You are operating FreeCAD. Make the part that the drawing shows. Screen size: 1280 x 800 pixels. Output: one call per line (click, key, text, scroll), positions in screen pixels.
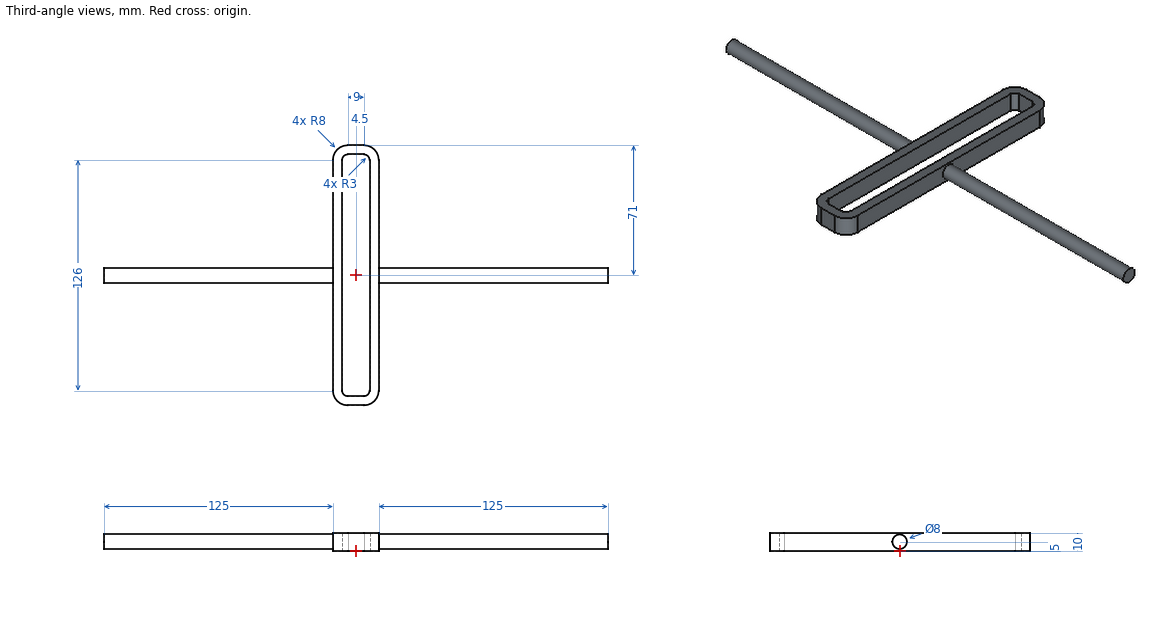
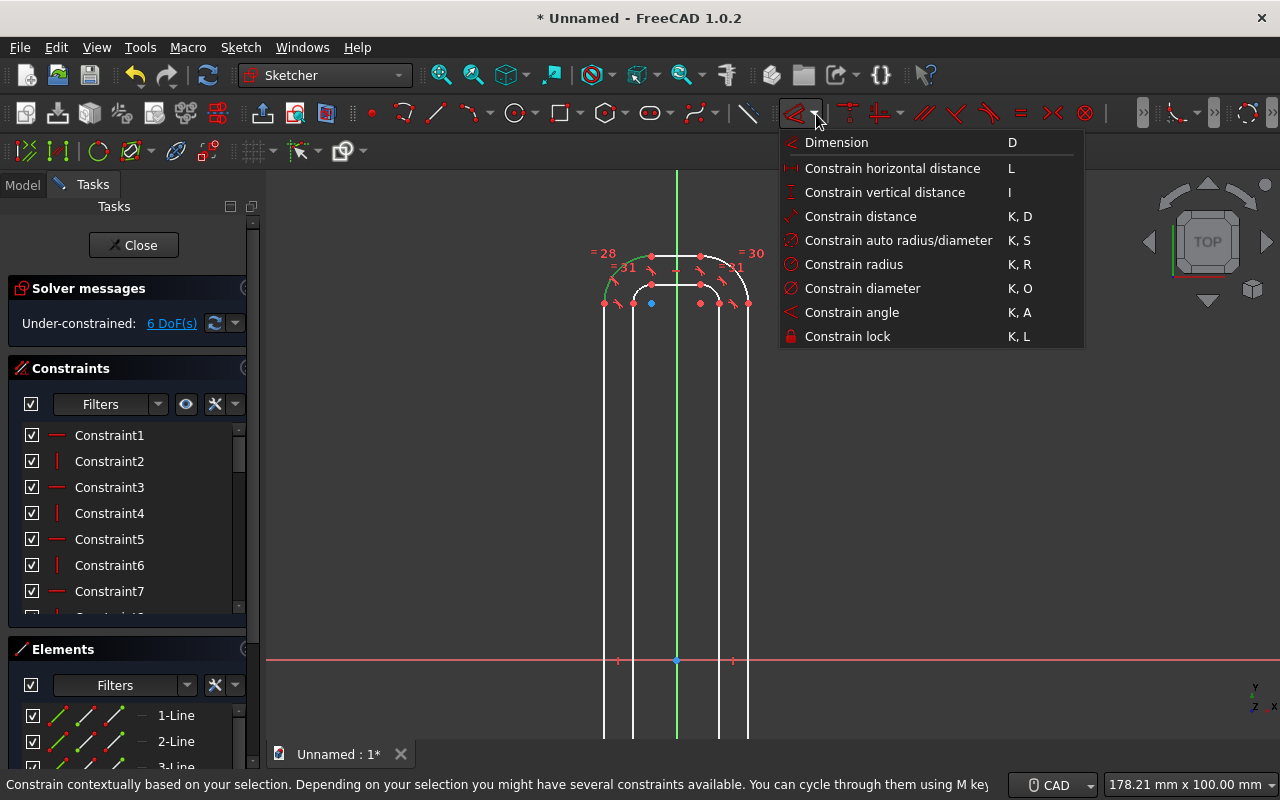
click(932, 264)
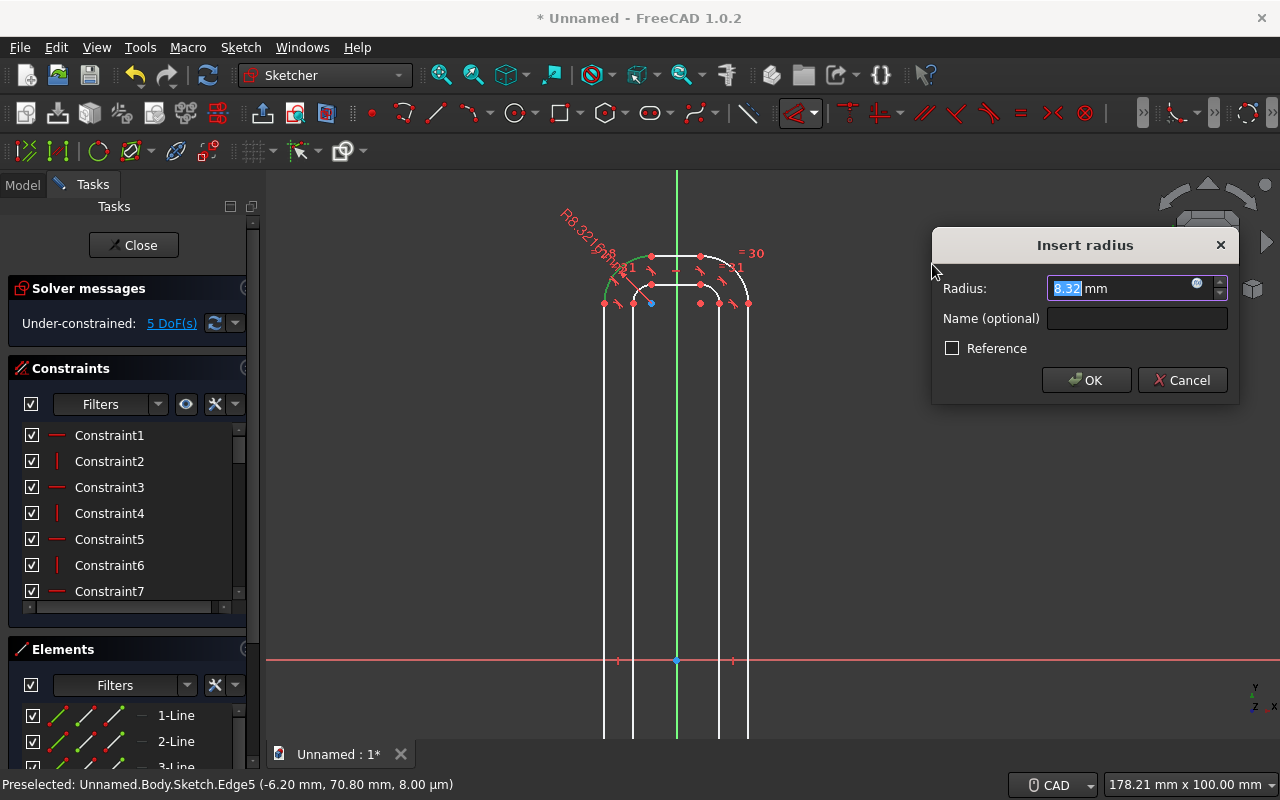
text(8)
key(Return)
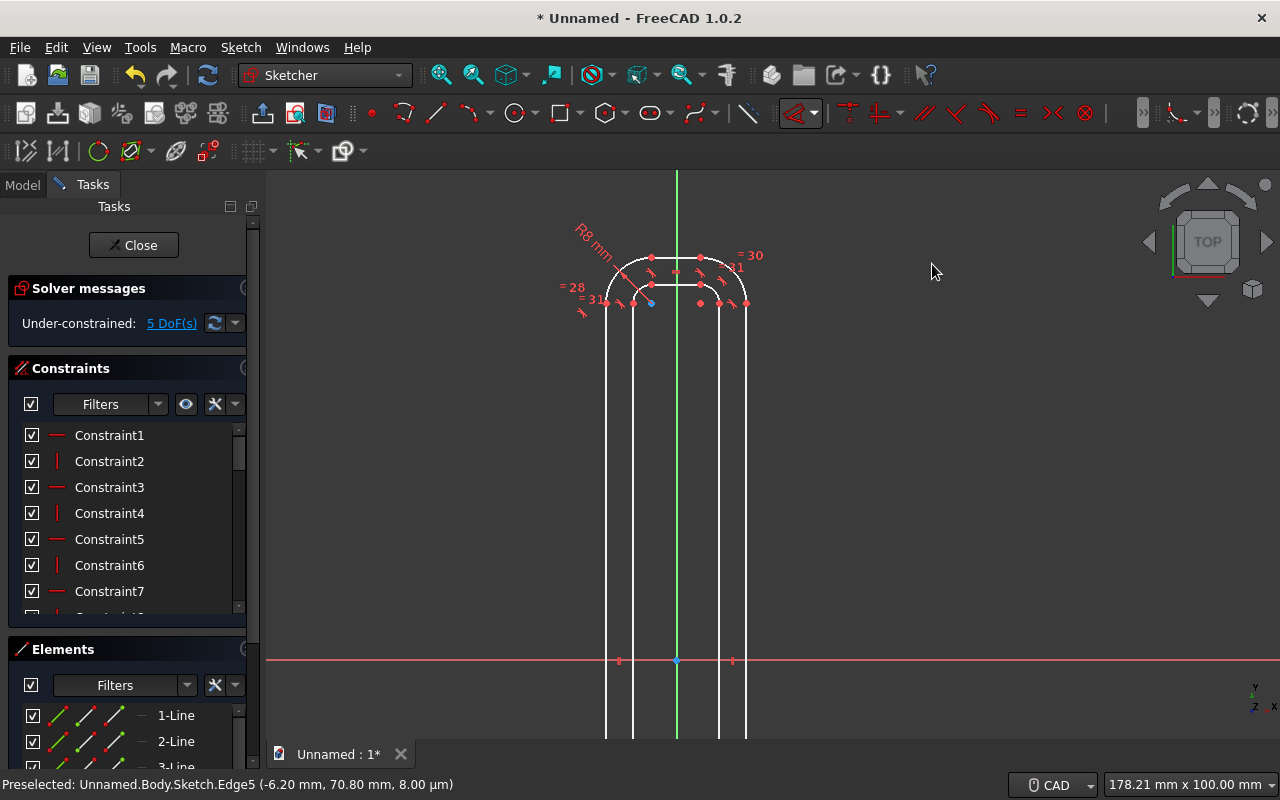
scroll(714, 290, up, 5)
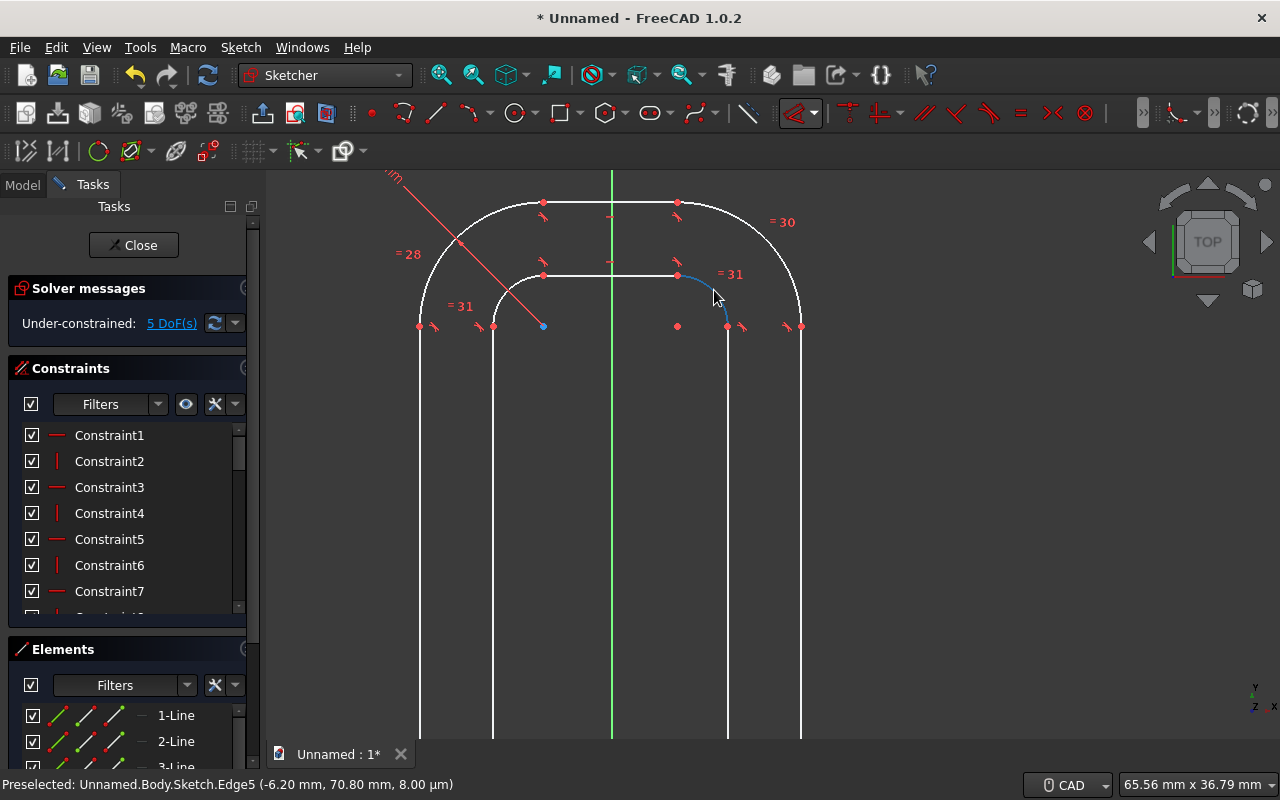
click(713, 291)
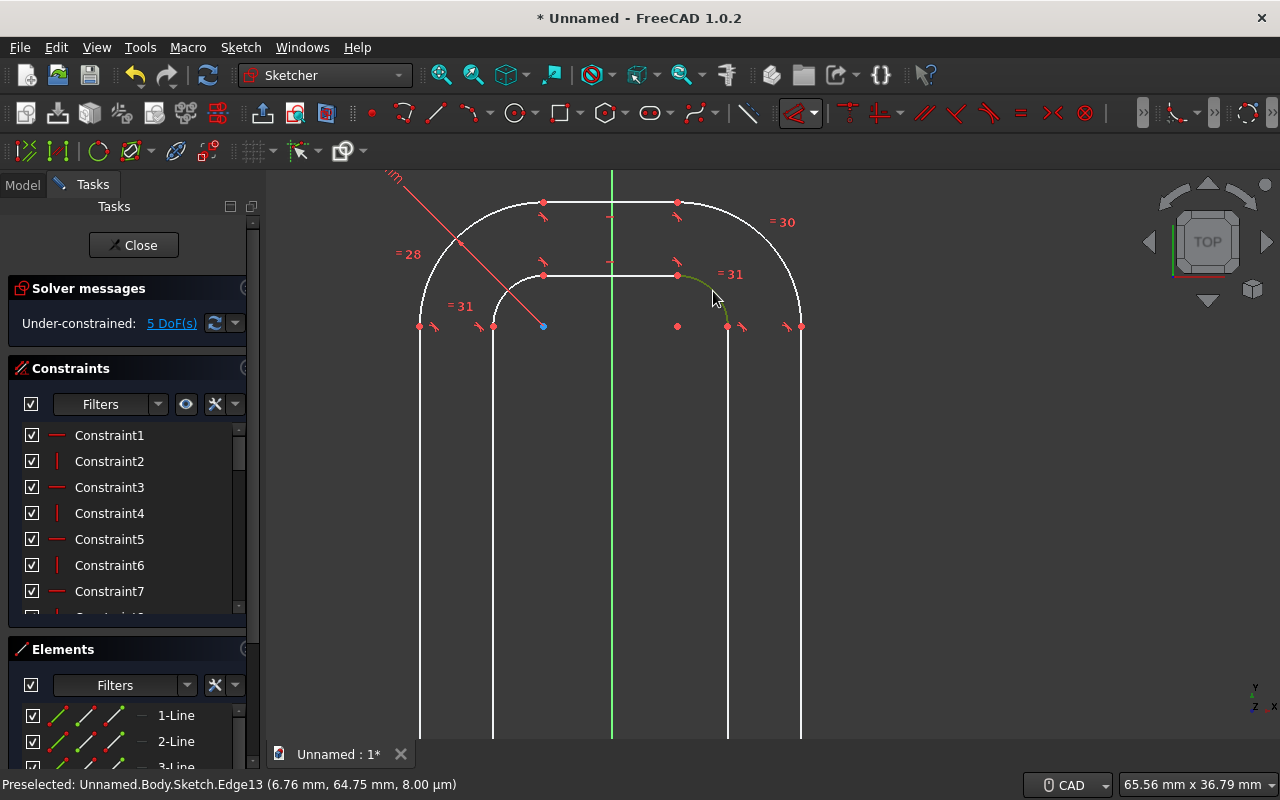
click(816, 114)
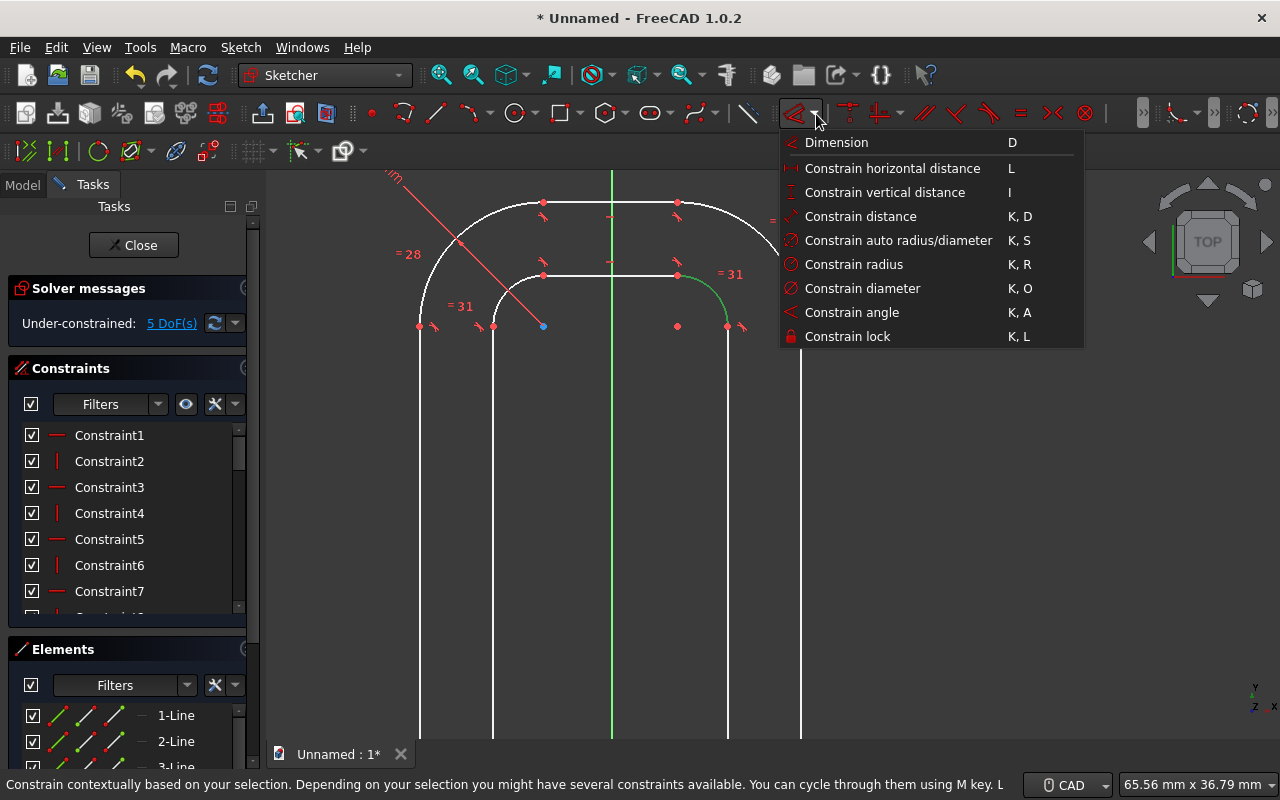
click(932, 264)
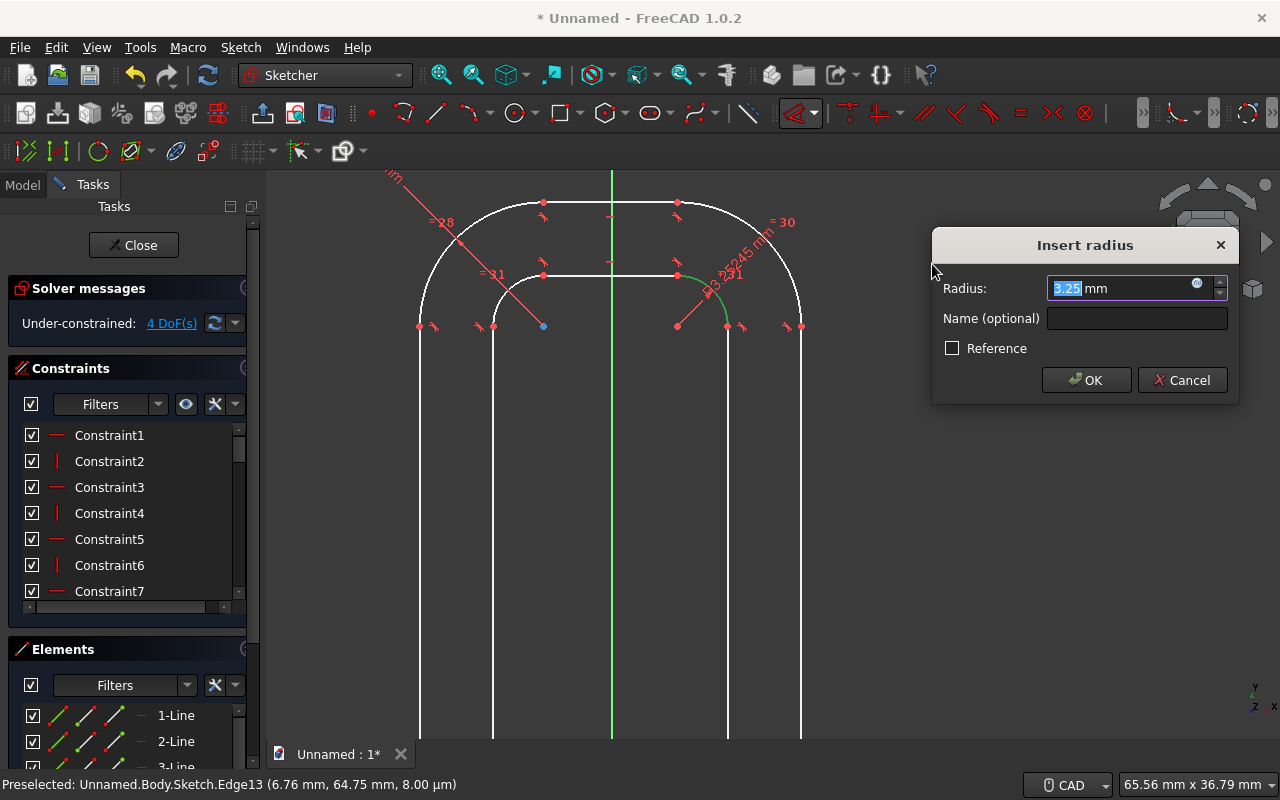
text(3)
key(Return)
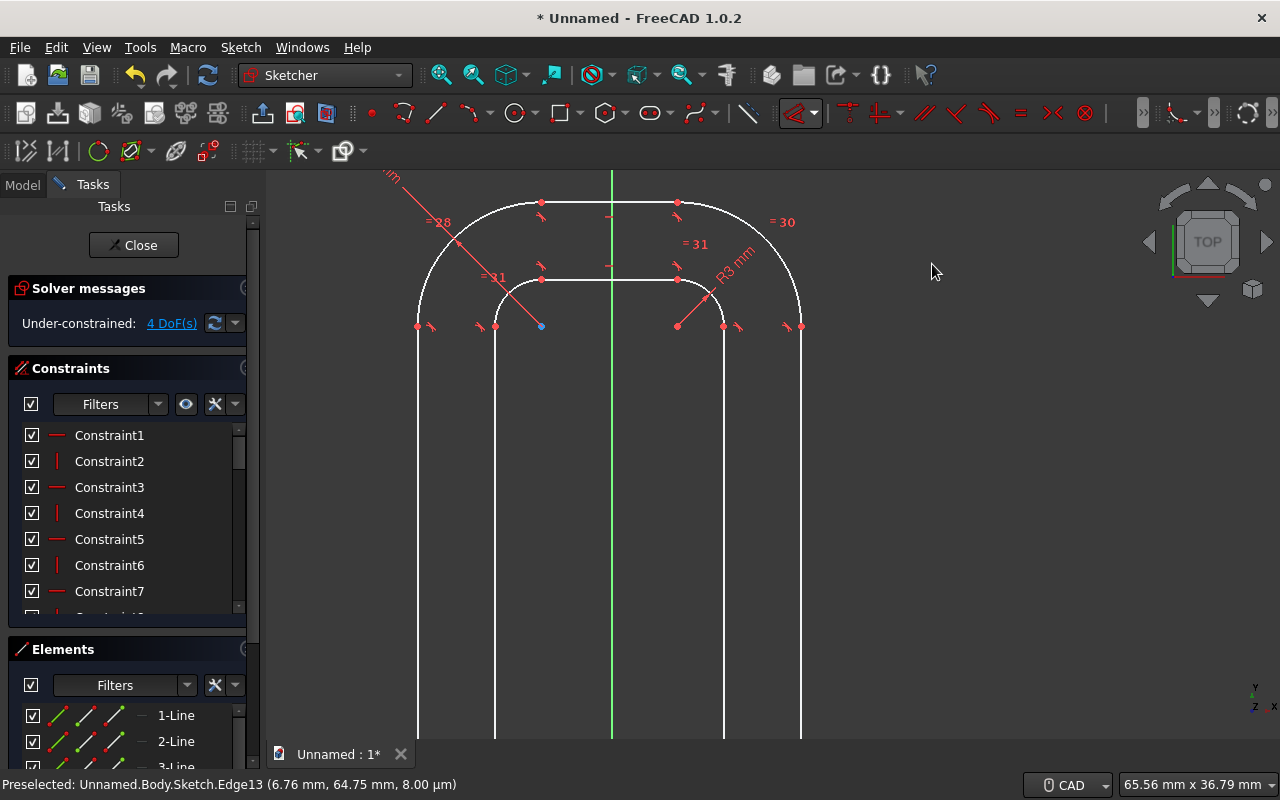
click(637, 202)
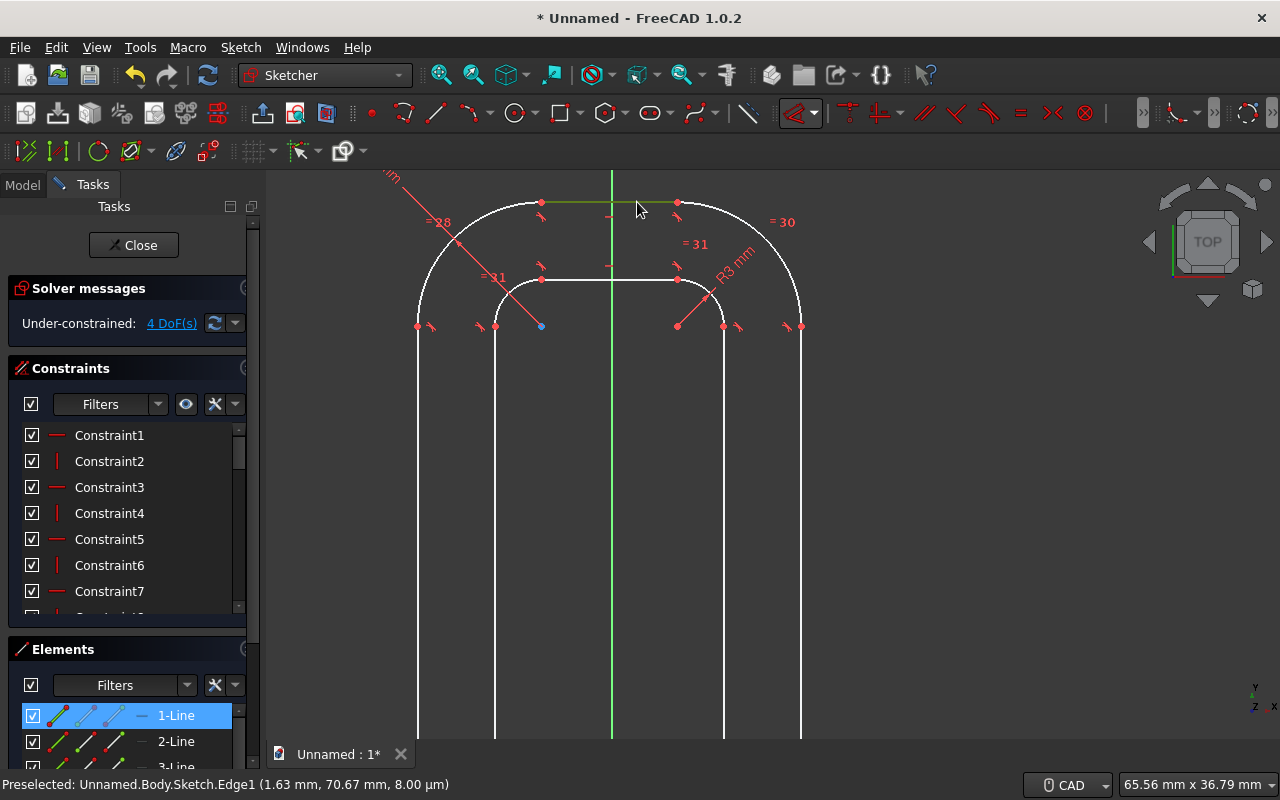
click(816, 114)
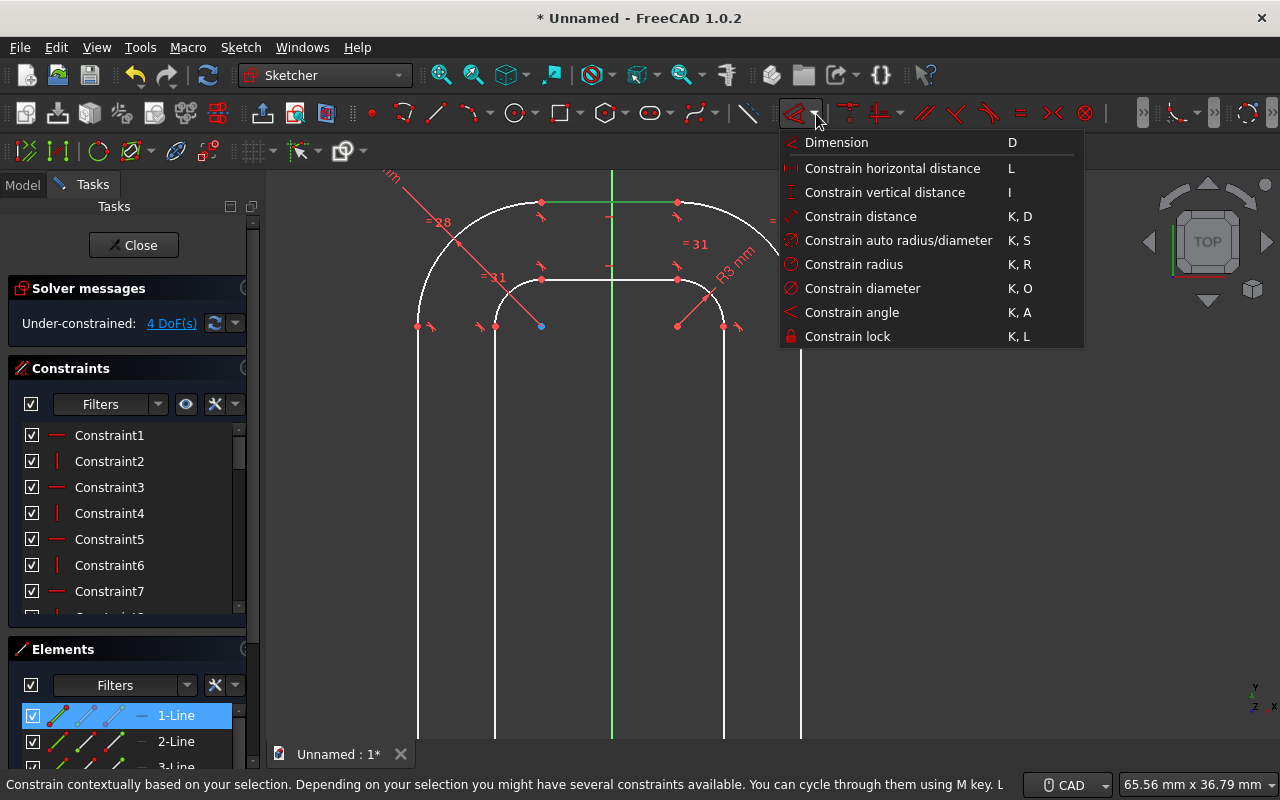
click(932, 168)